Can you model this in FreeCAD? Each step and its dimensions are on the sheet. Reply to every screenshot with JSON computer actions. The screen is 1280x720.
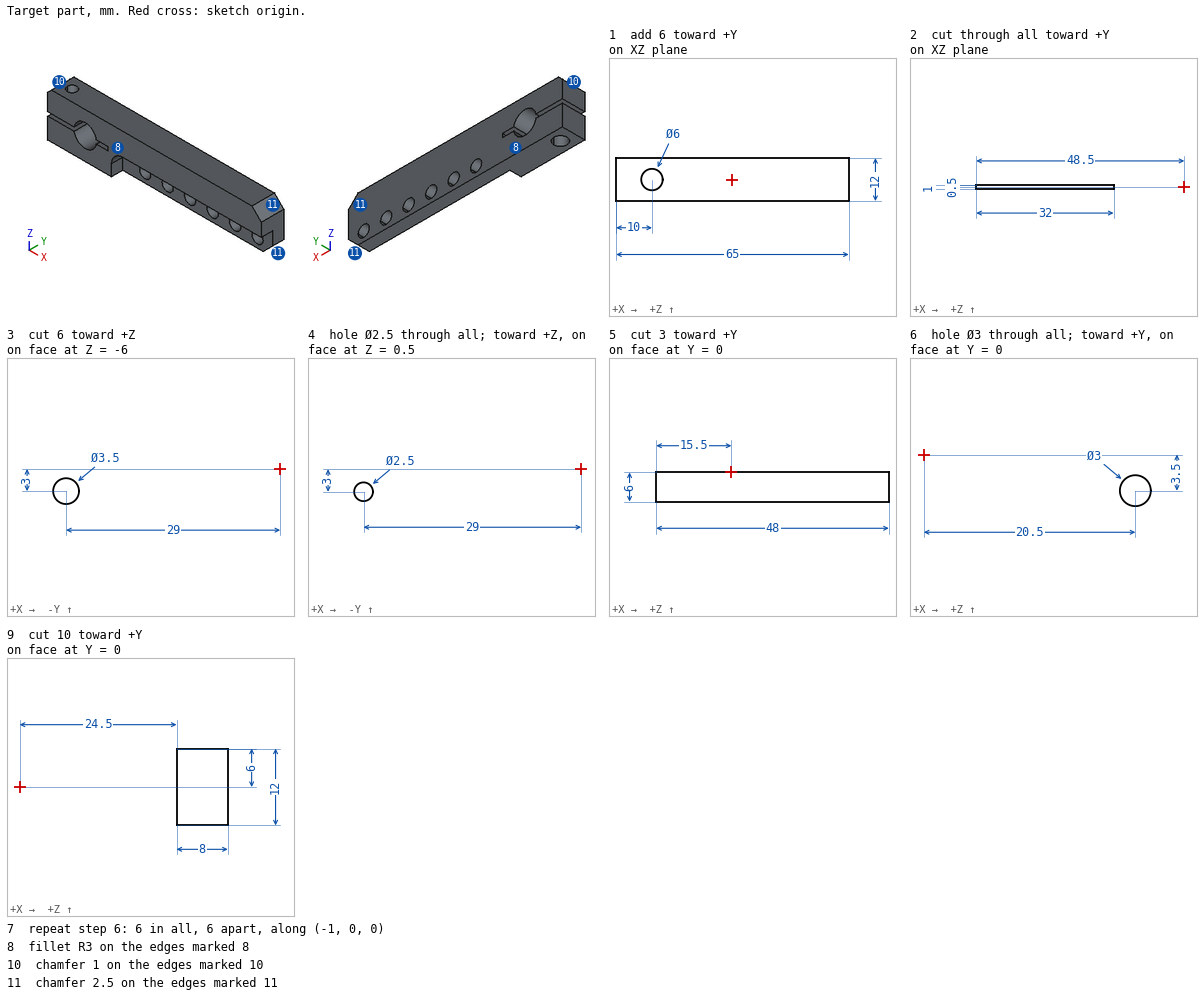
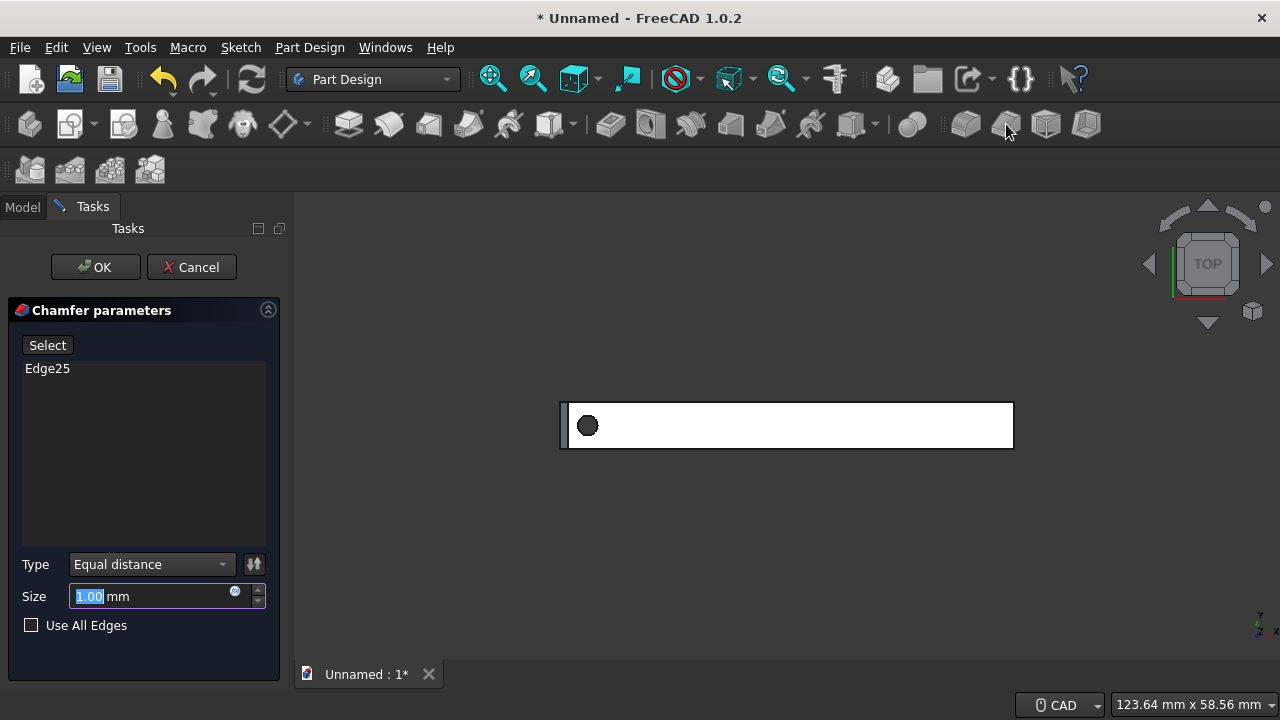
{"action": "type", "text": "1"}
{"action": "key", "text": "Tab"}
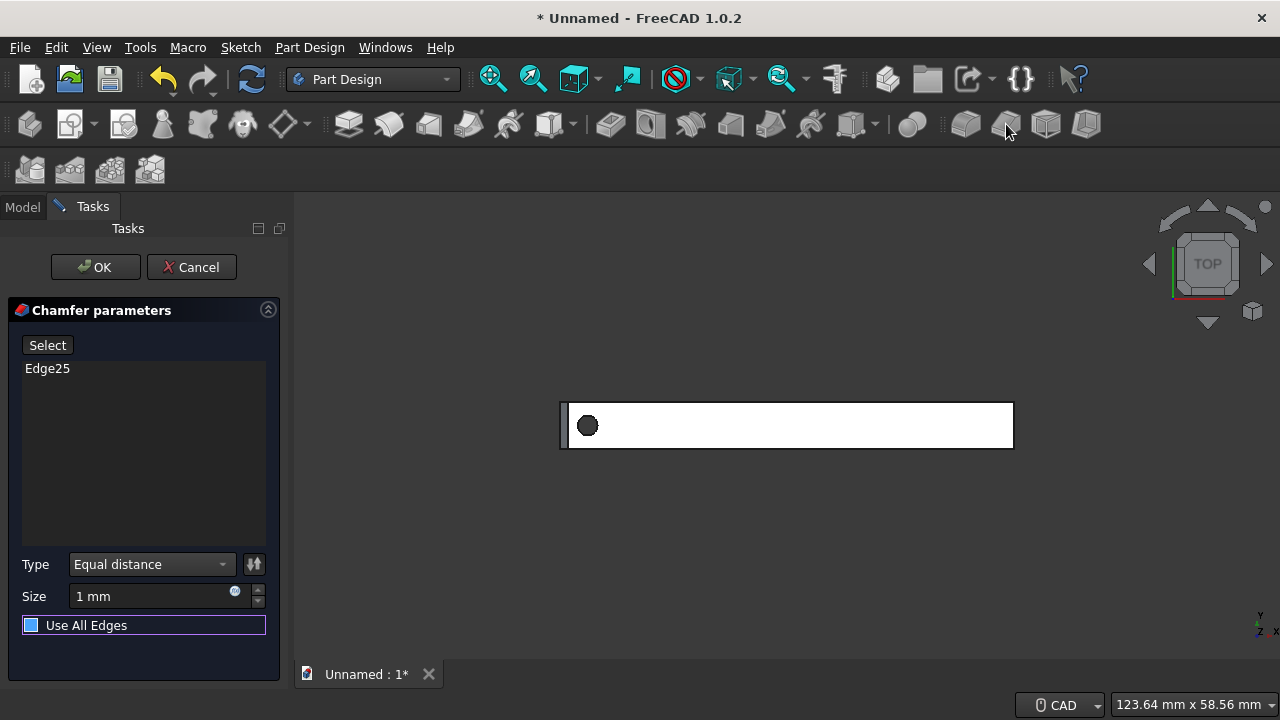
{"action": "left_click", "coordinate": [96, 267]}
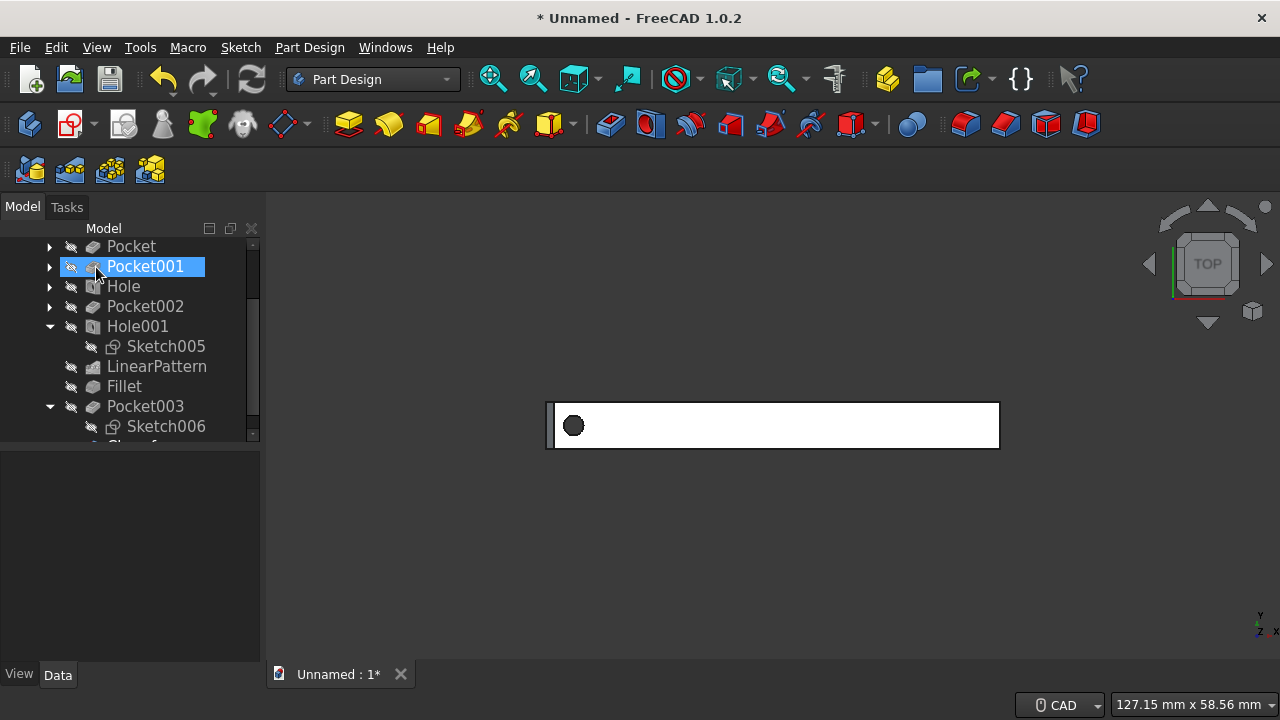
{"action": "left_click", "coordinate": [494, 80]}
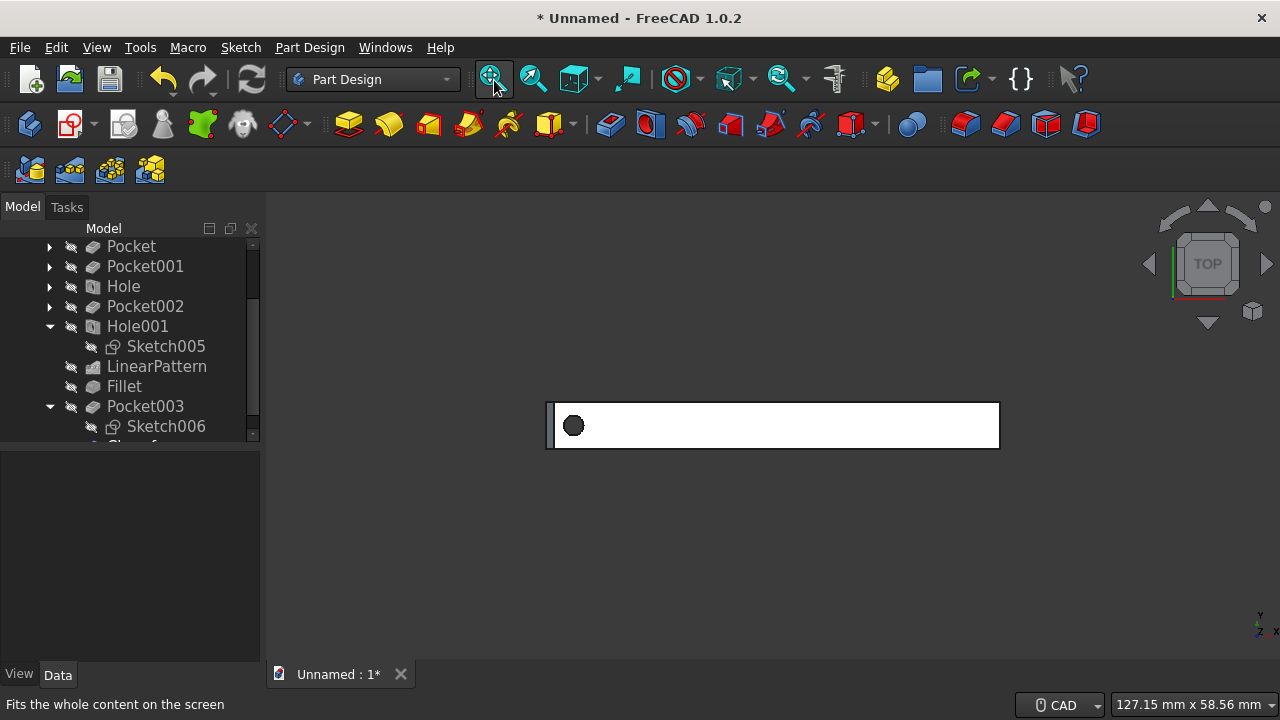
{"action": "left_click", "coordinate": [1000, 424]}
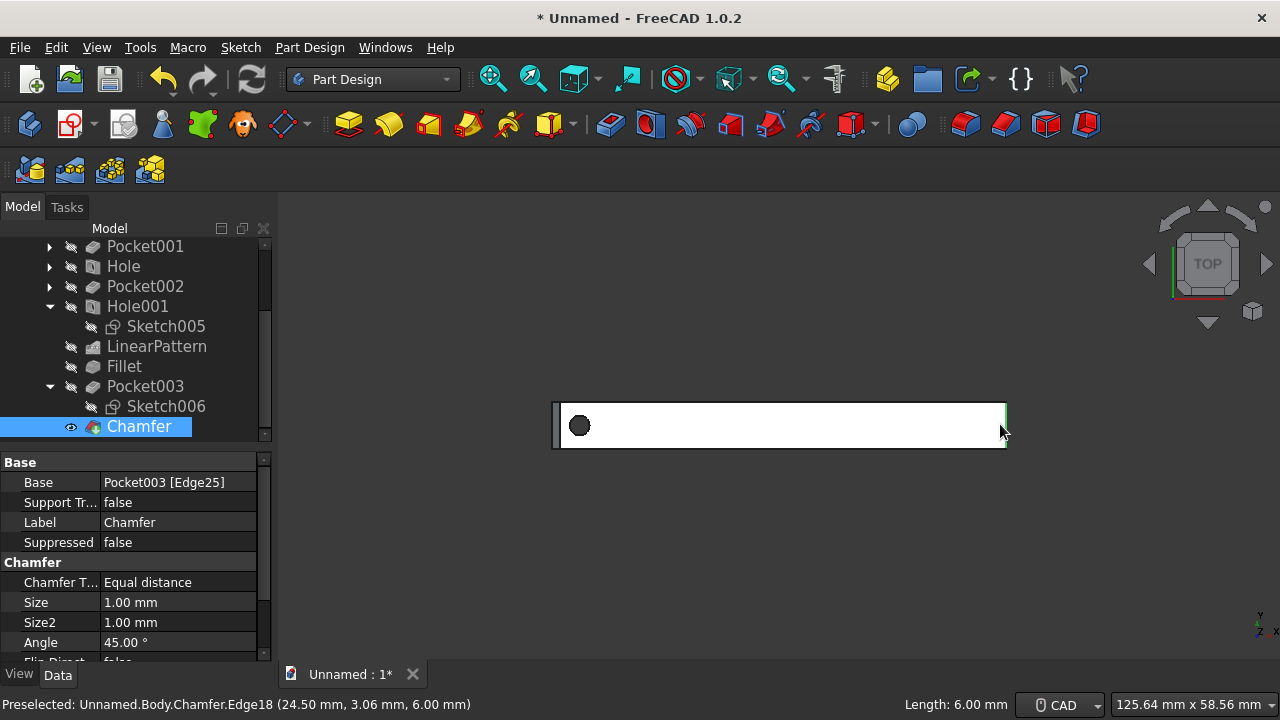
{"action": "key", "text": "0"}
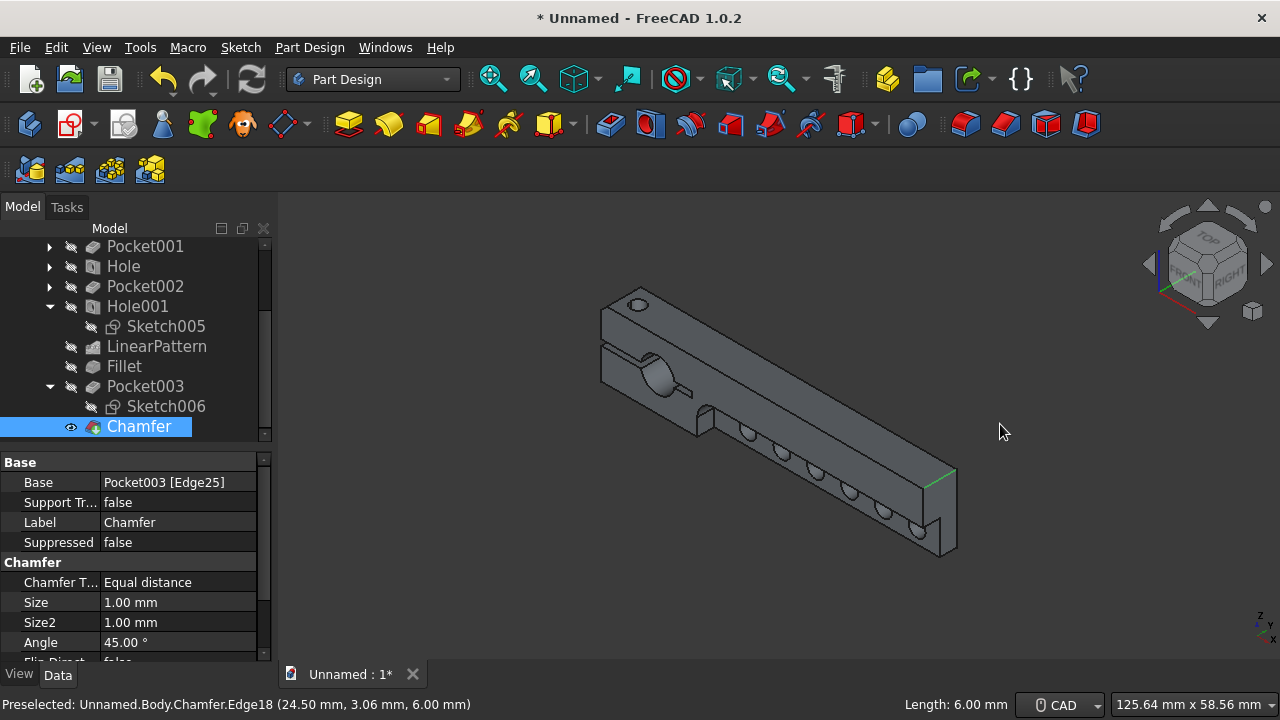
{"action": "key", "text": "2"}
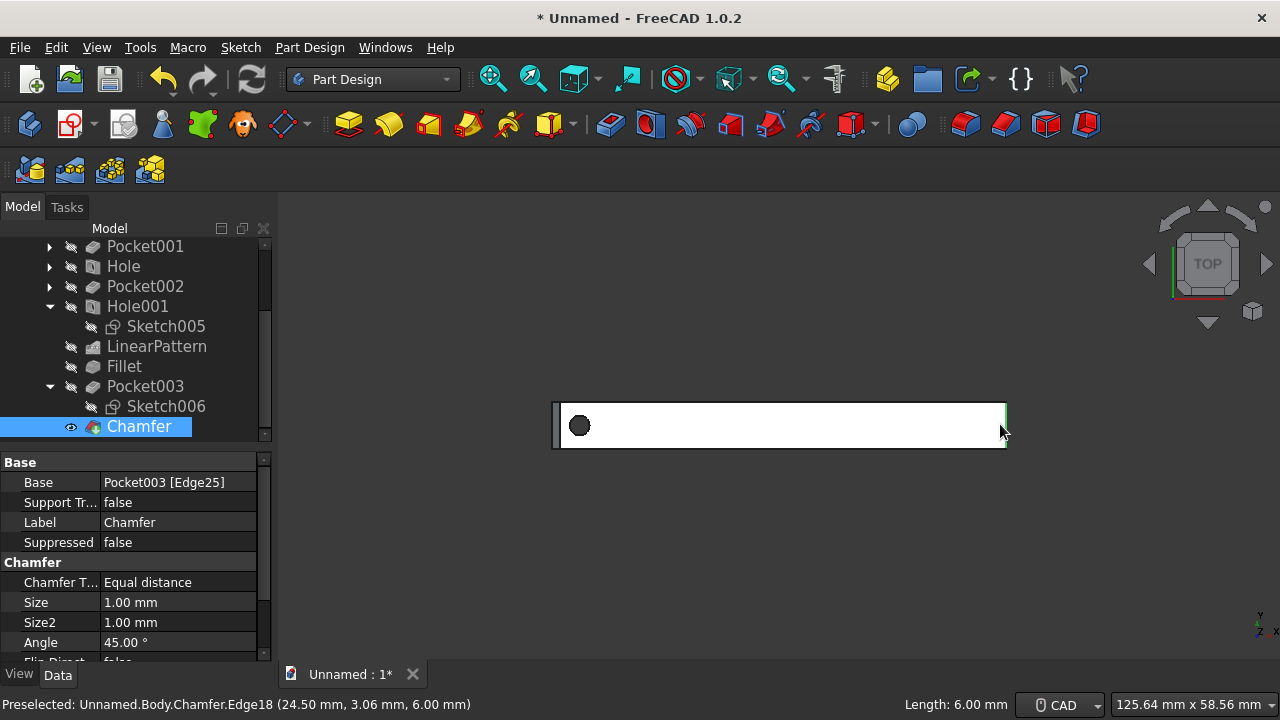
{"action": "key", "text": "1"}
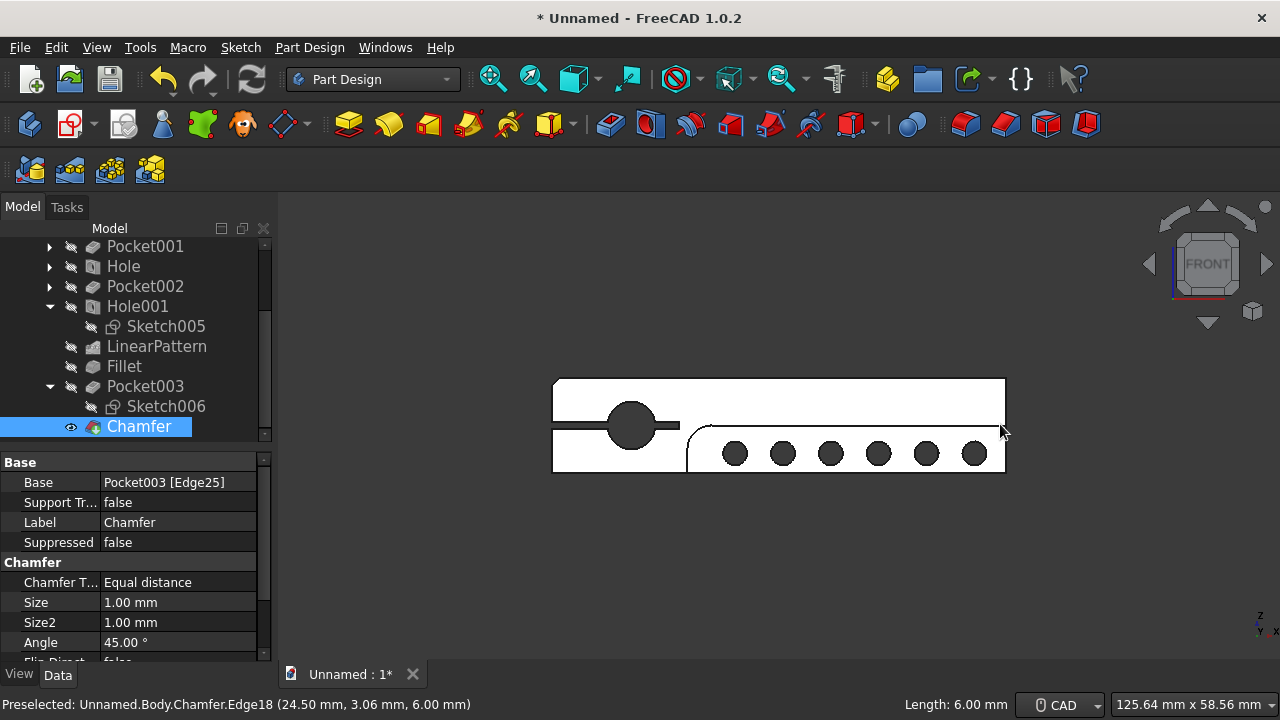
{"action": "key", "text": "3"}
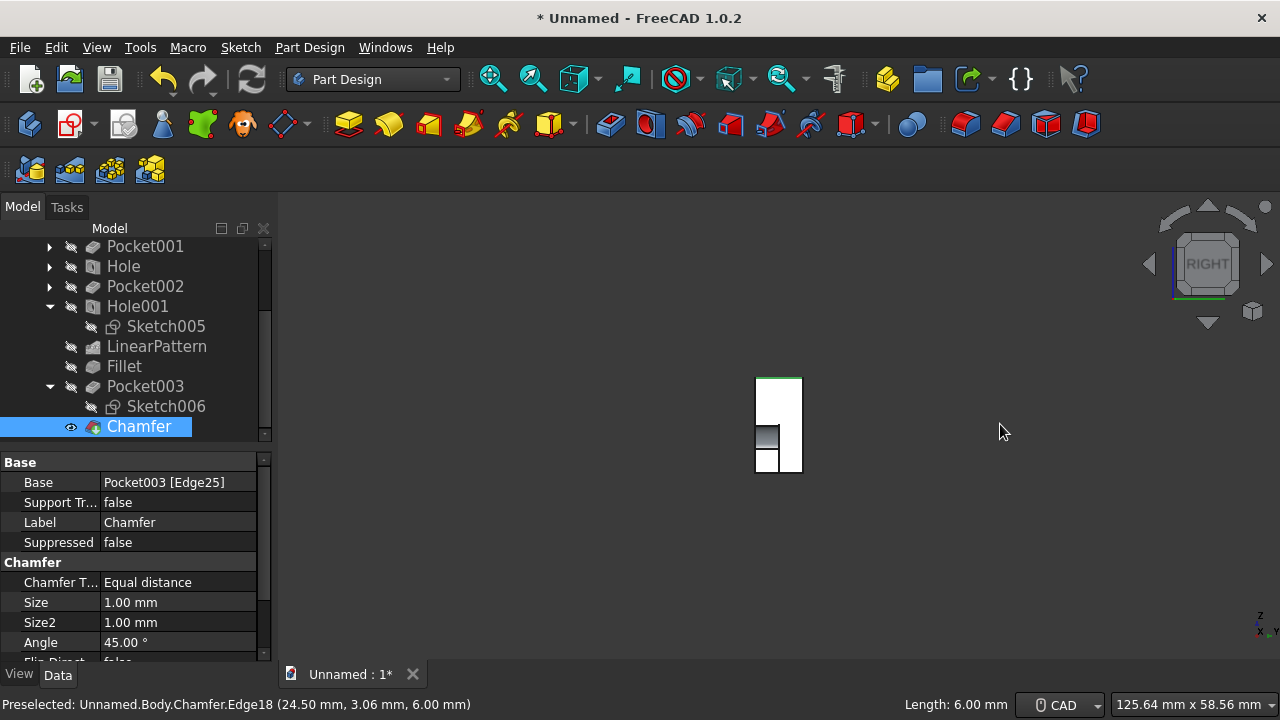
{"action": "key", "text": "v f"}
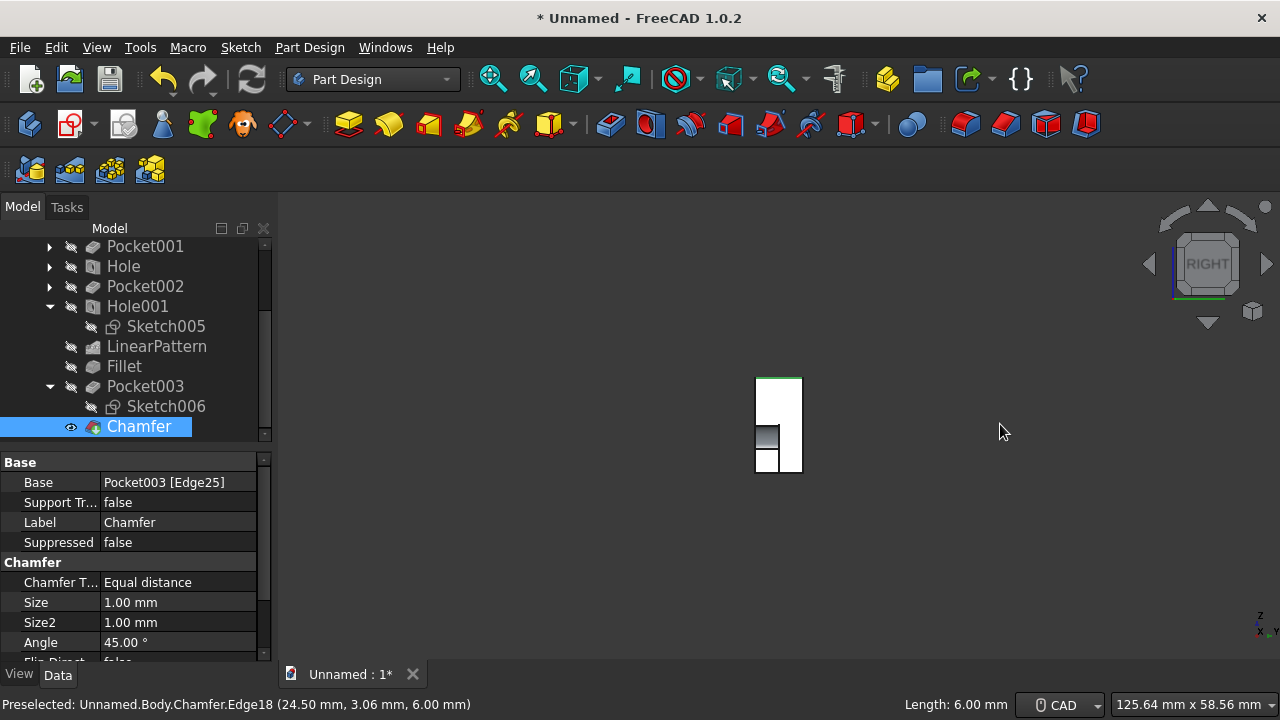
{"action": "left_click", "coordinate": [791, 472], "text": "ctrl"}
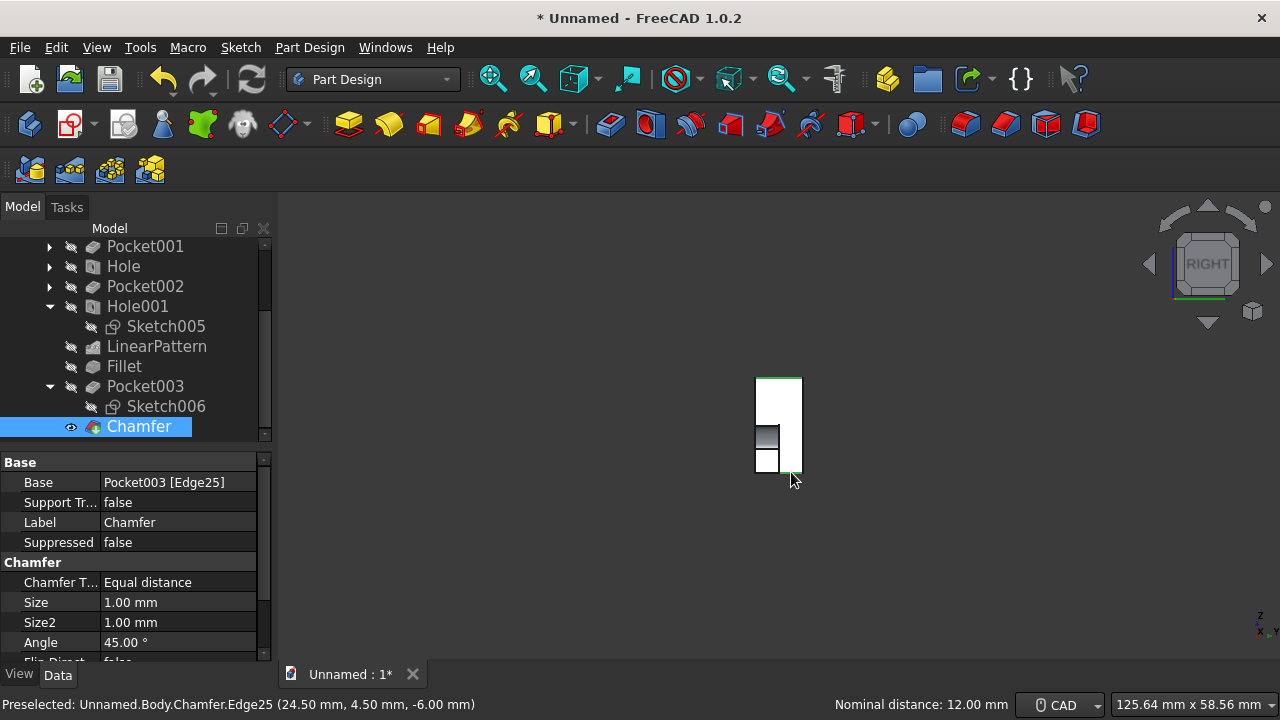
{"action": "left_click", "coordinate": [1006, 124]}